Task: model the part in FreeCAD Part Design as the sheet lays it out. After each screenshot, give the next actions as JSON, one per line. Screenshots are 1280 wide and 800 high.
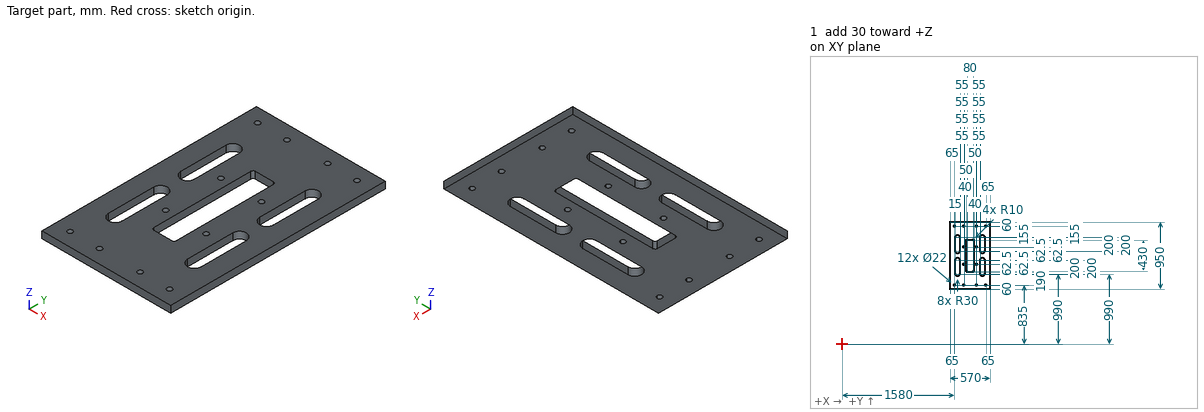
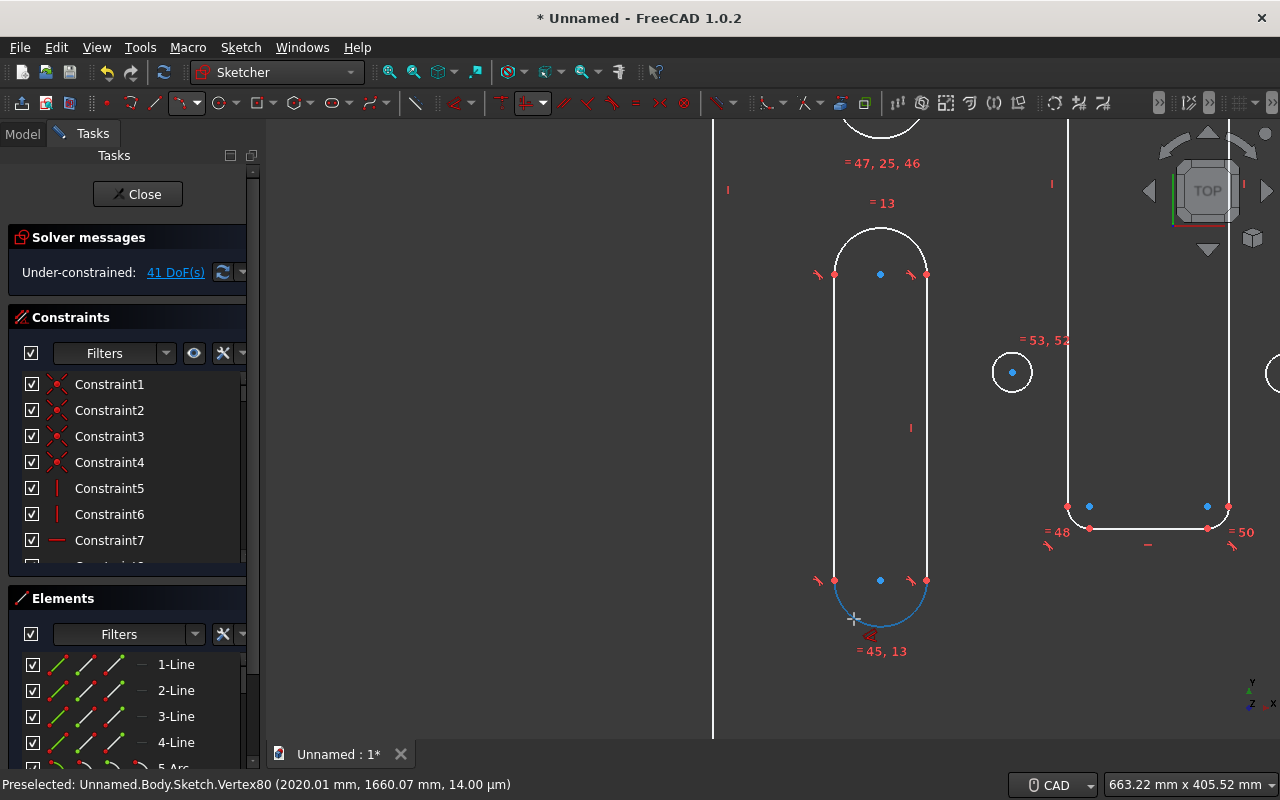
{"action": "left_click", "coordinate": [854, 618]}
{"action": "left_click", "coordinate": [835, 644]}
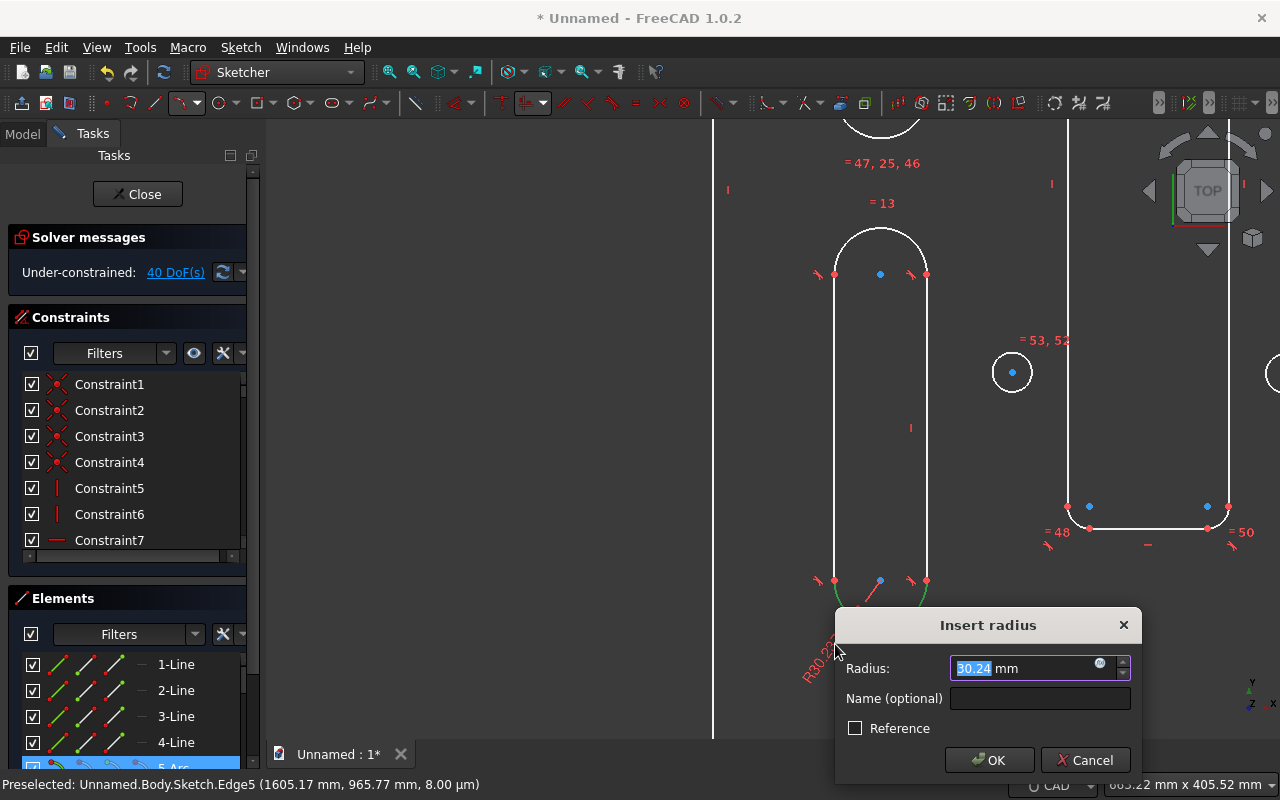
{"action": "type", "text": "30"}
{"action": "key", "text": "Return"}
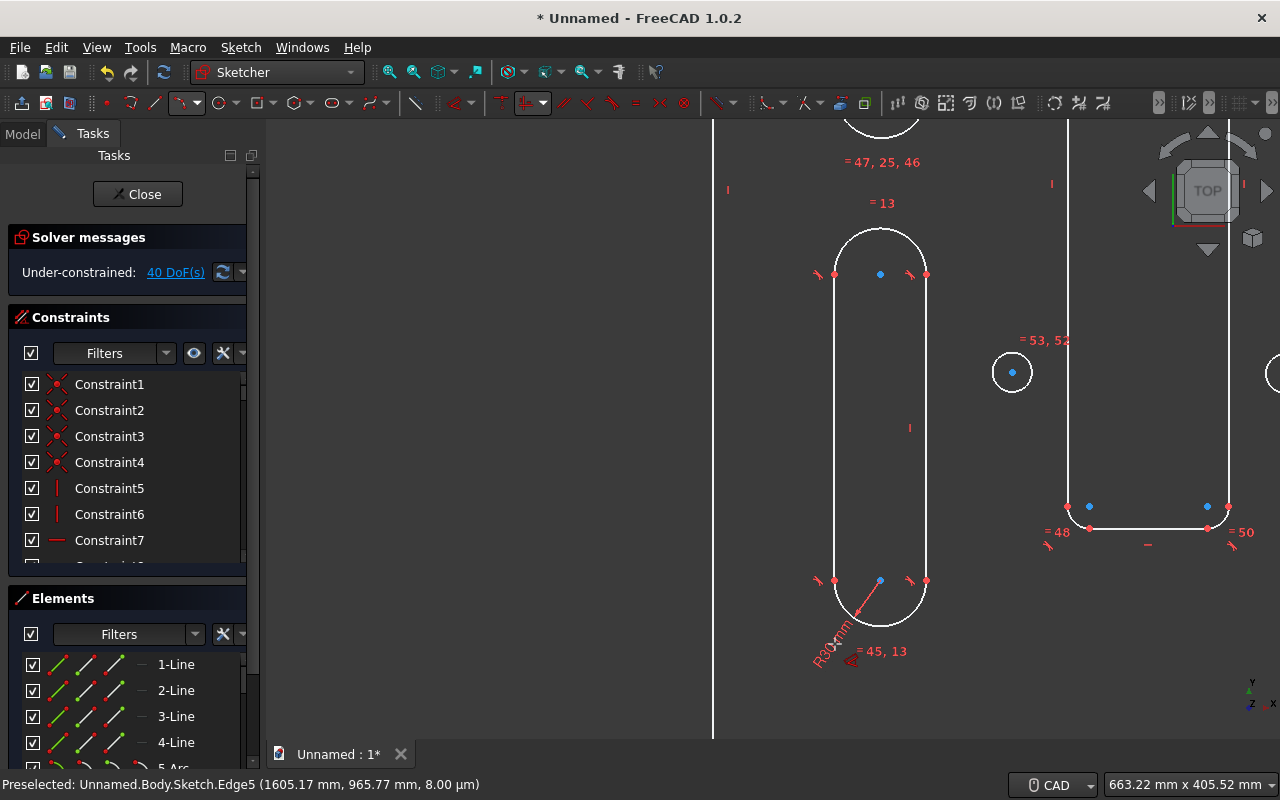
{"action": "scroll", "coordinate": [1070, 517], "scroll_direction": "up", "scroll_amount": 5}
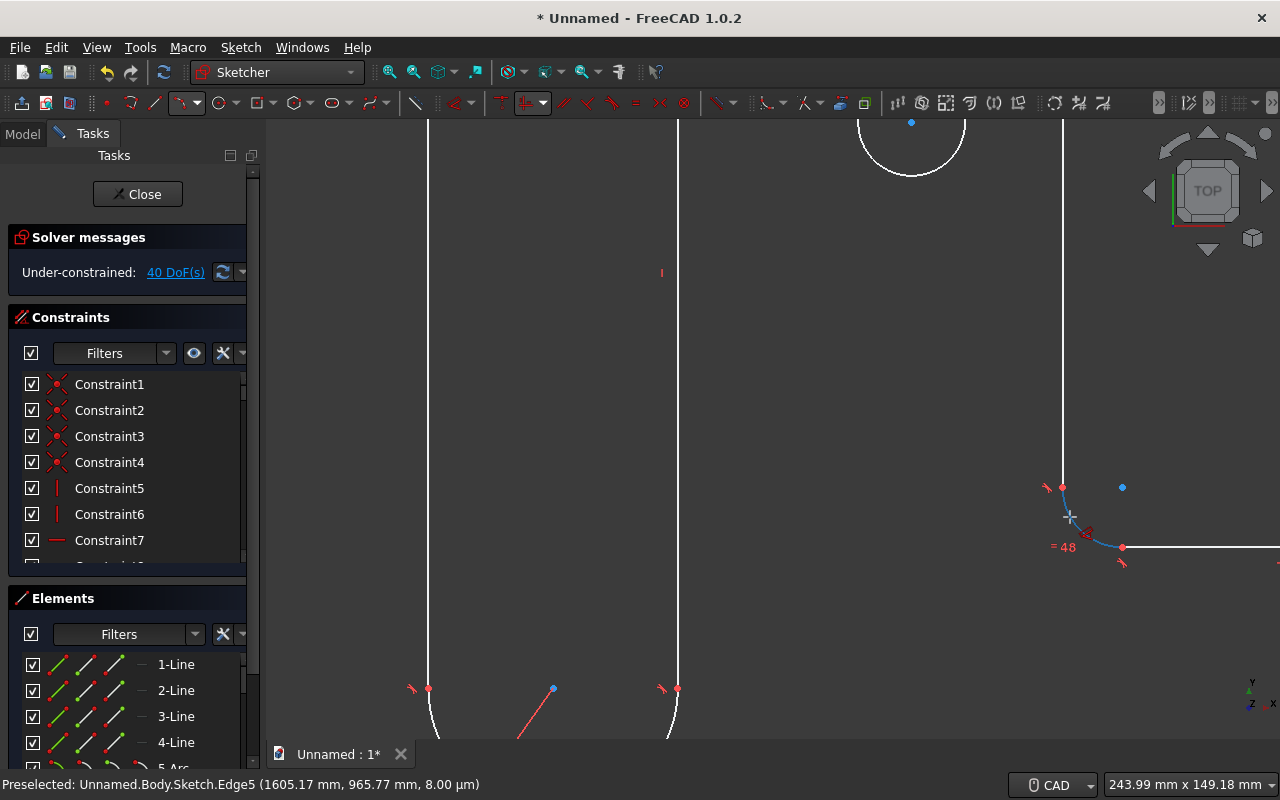
{"action": "left_click", "coordinate": [1069, 515]}
{"action": "left_click", "coordinate": [1041, 530]}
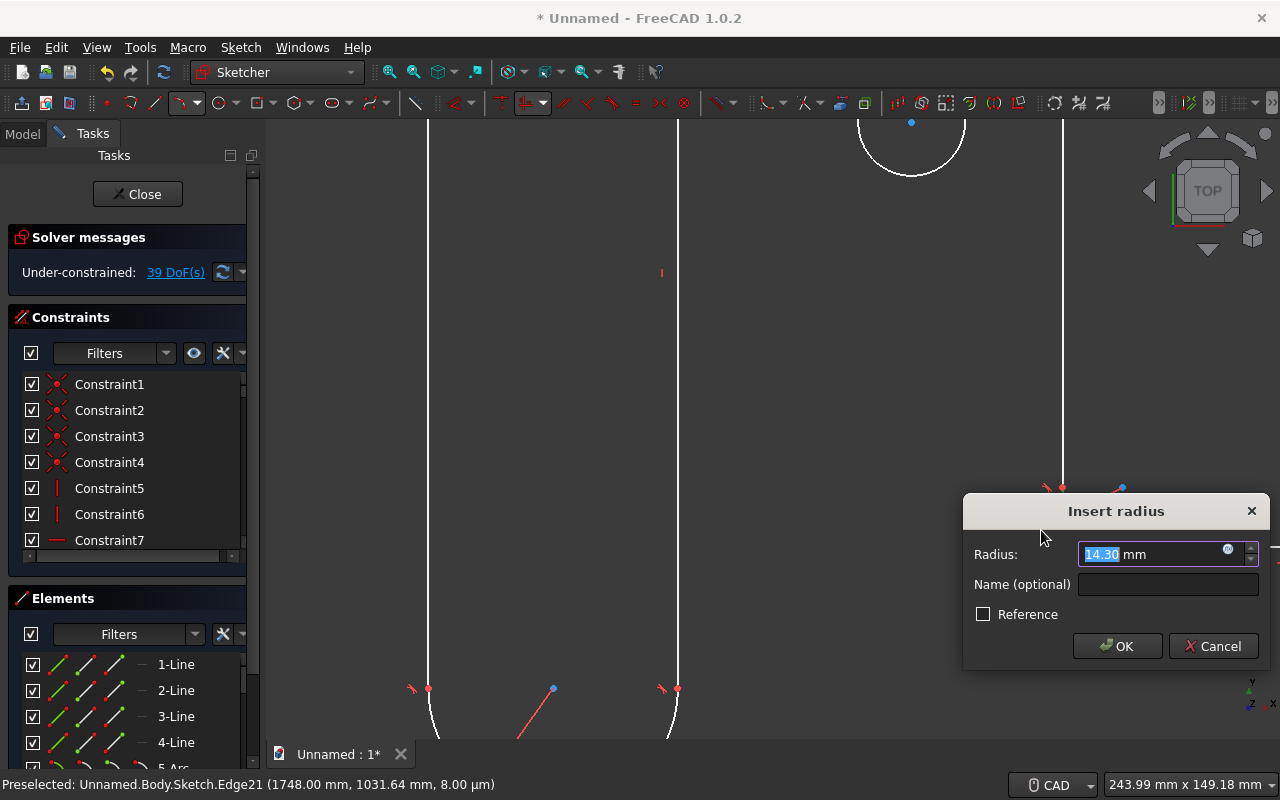
{"action": "type", "text": "10"}
{"action": "key", "text": "Return"}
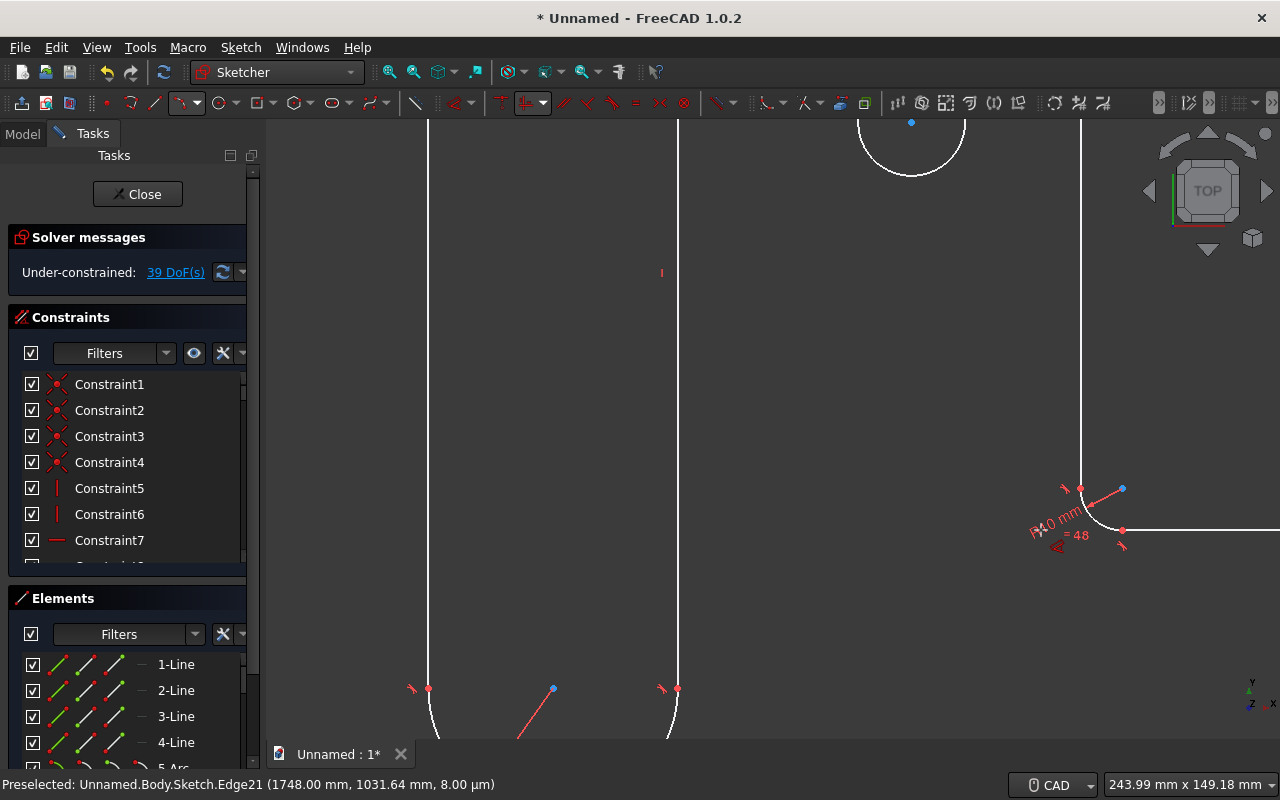
{"action": "scroll", "coordinate": [871, 378], "scroll_direction": "down", "scroll_amount": 14}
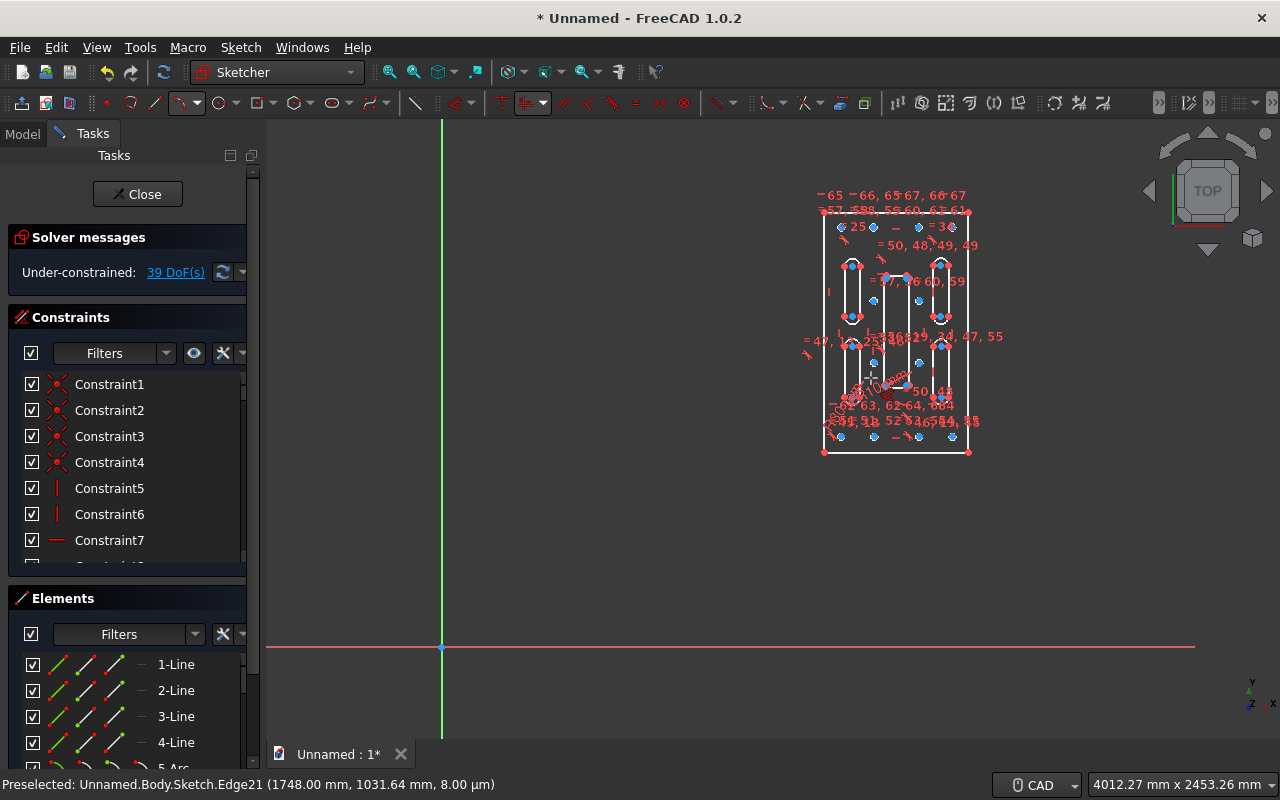
{"action": "scroll", "coordinate": [843, 435], "scroll_direction": "up", "scroll_amount": 10}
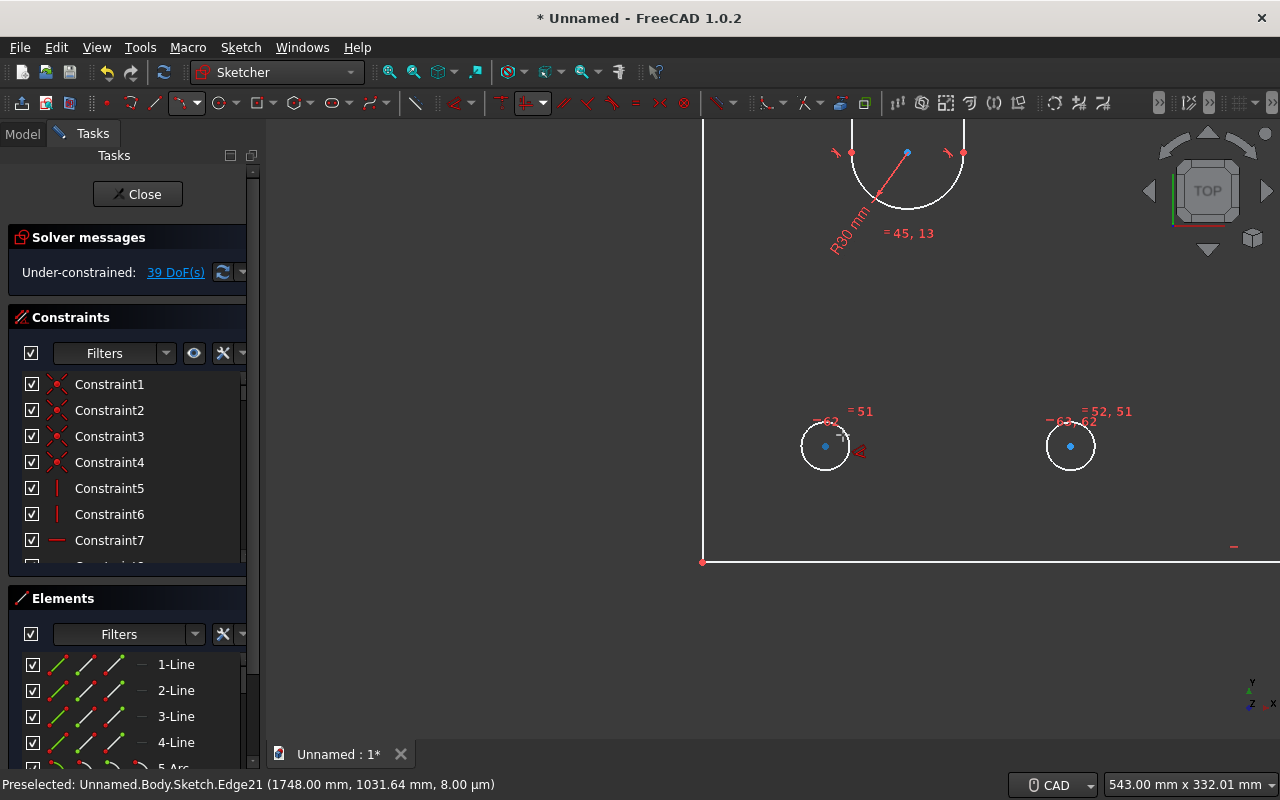
{"action": "left_click", "coordinate": [842, 429]}
{"action": "left_click", "coordinate": [864, 406]}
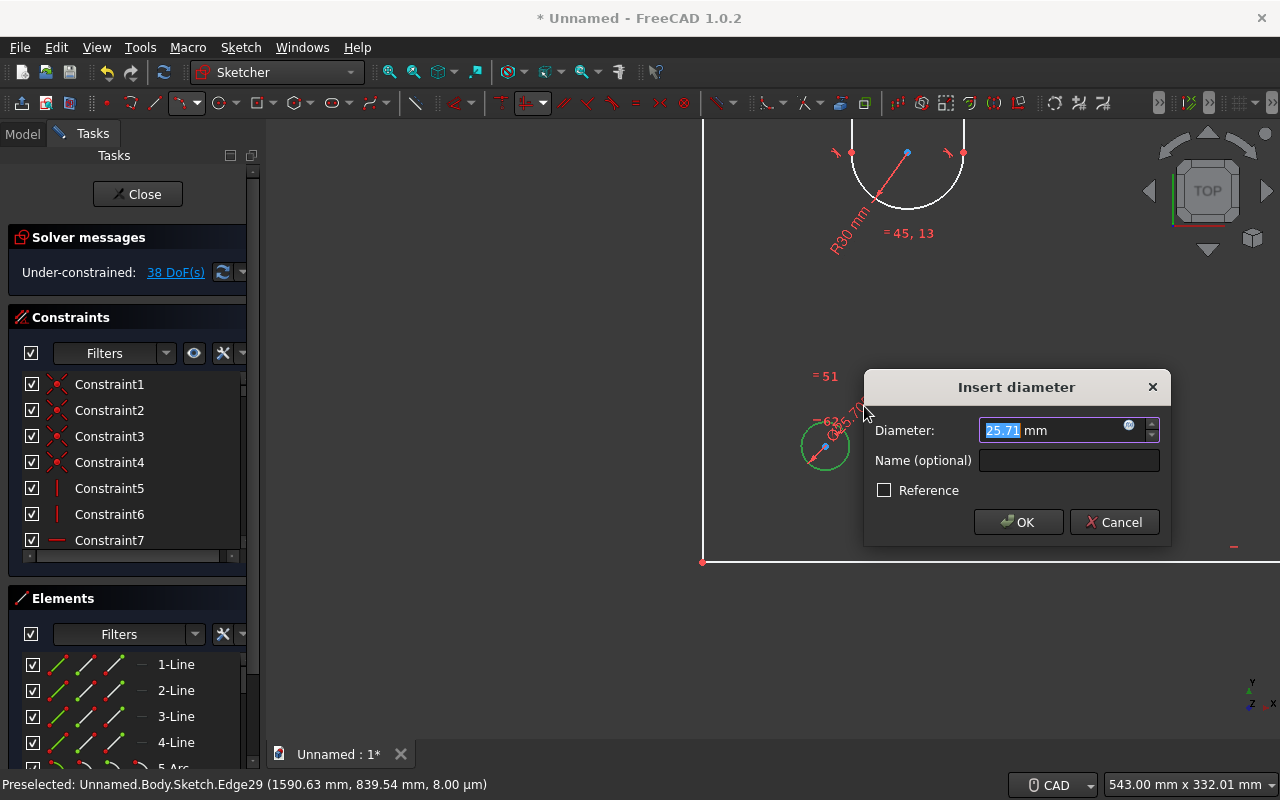
{"action": "type", "text": "22"}
{"action": "key", "text": "Return"}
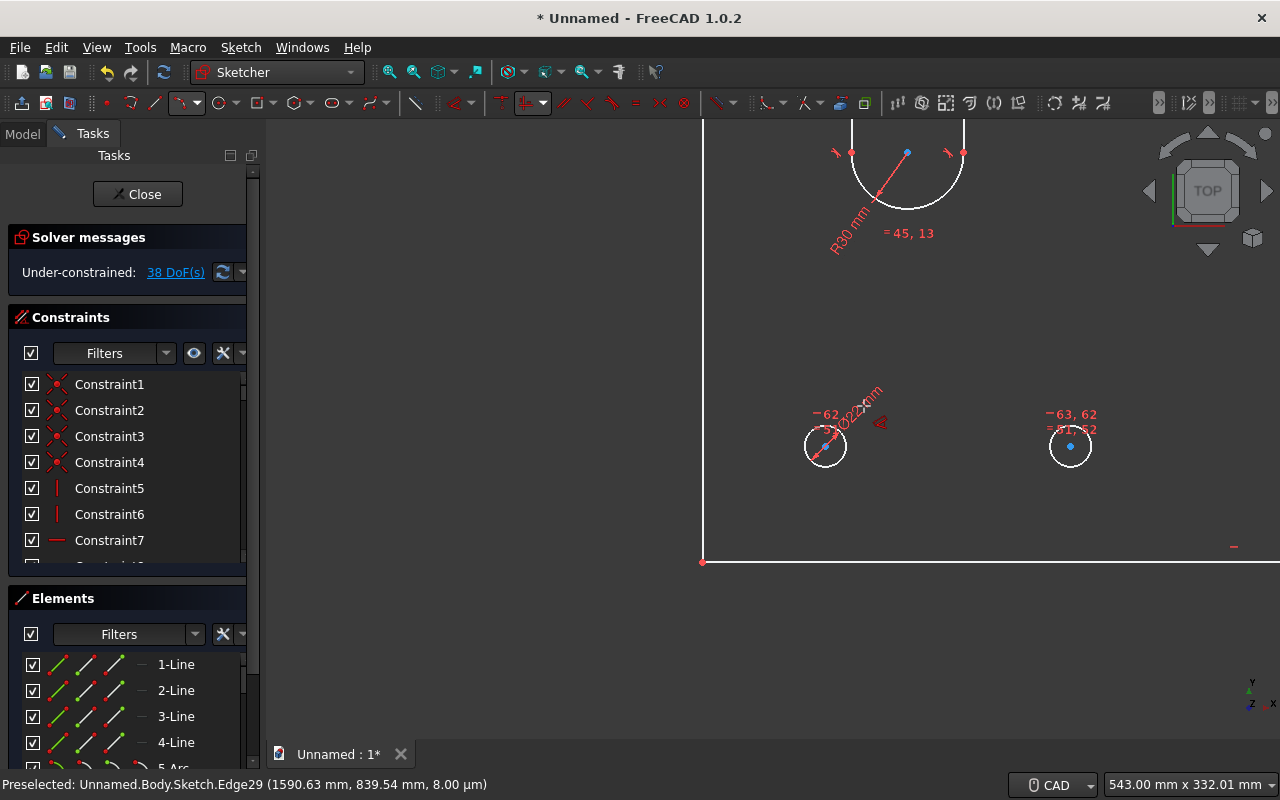
{"action": "scroll", "coordinate": [843, 435], "scroll_direction": "down", "scroll_amount": 10}